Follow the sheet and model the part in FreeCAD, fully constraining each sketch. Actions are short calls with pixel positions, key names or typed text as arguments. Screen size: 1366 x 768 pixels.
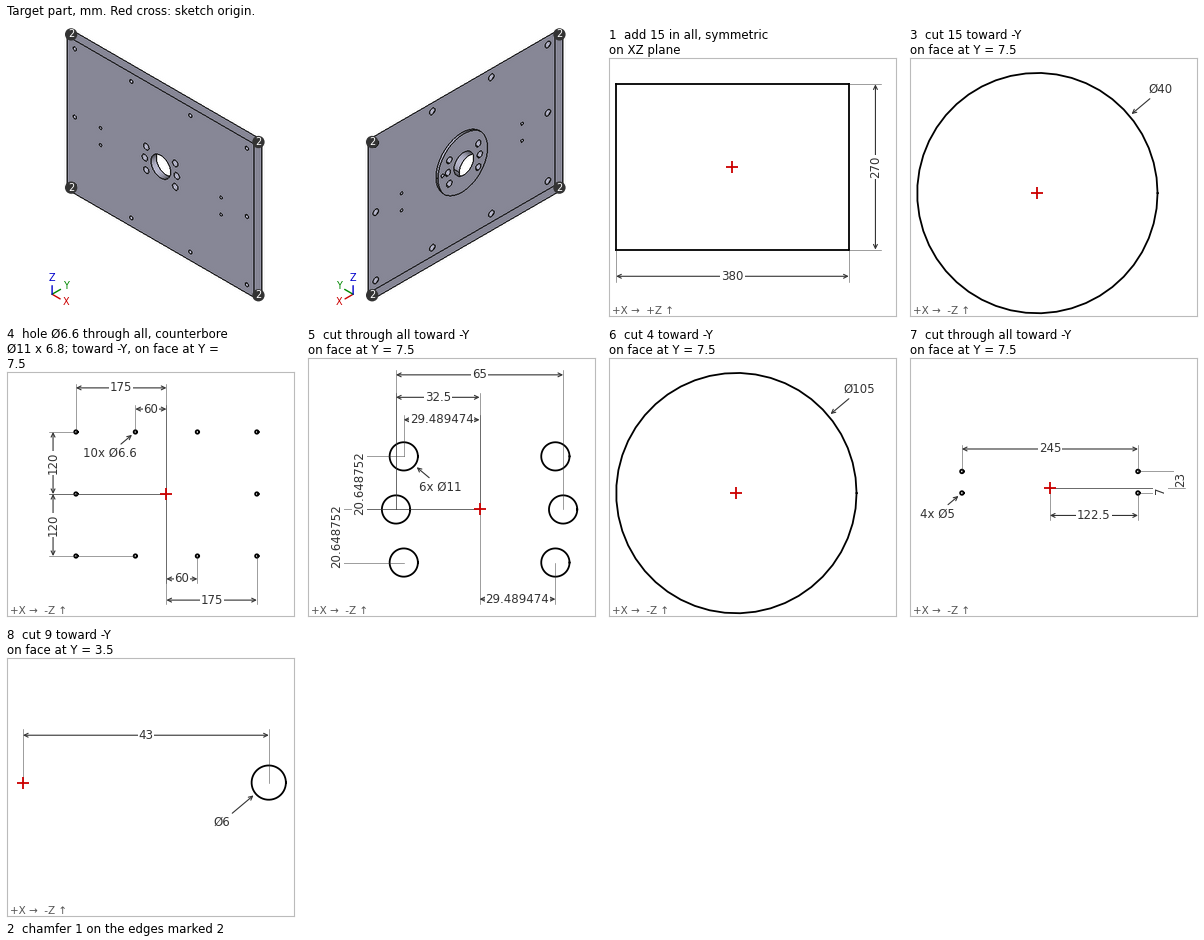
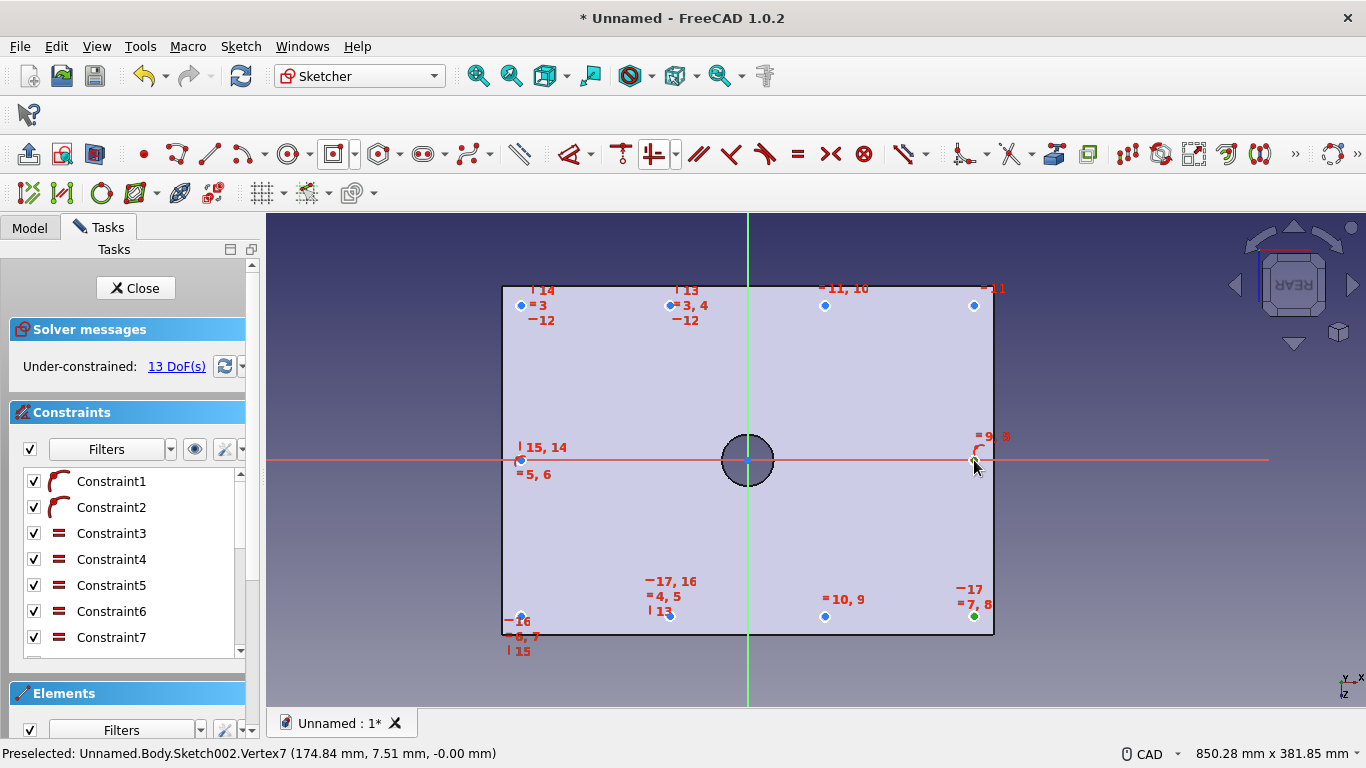
click(676, 154)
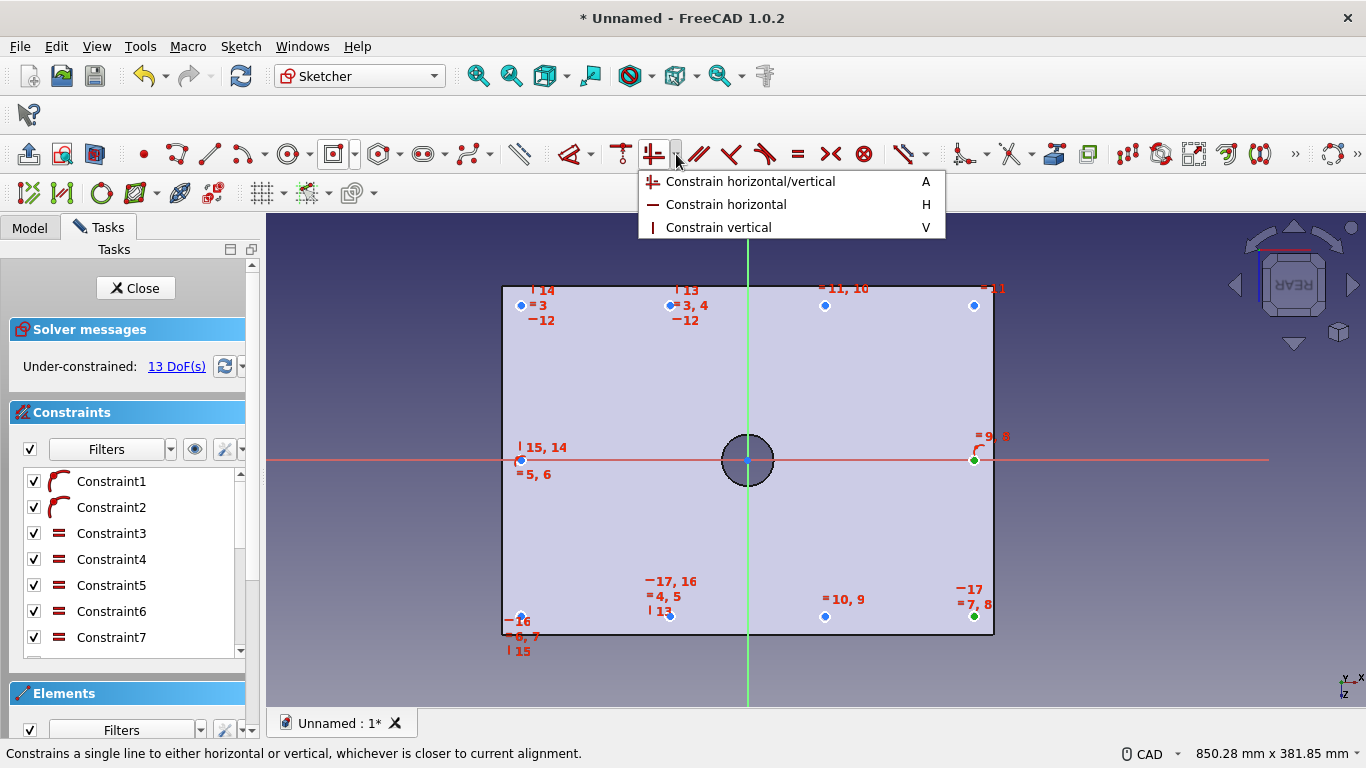
click(792, 228)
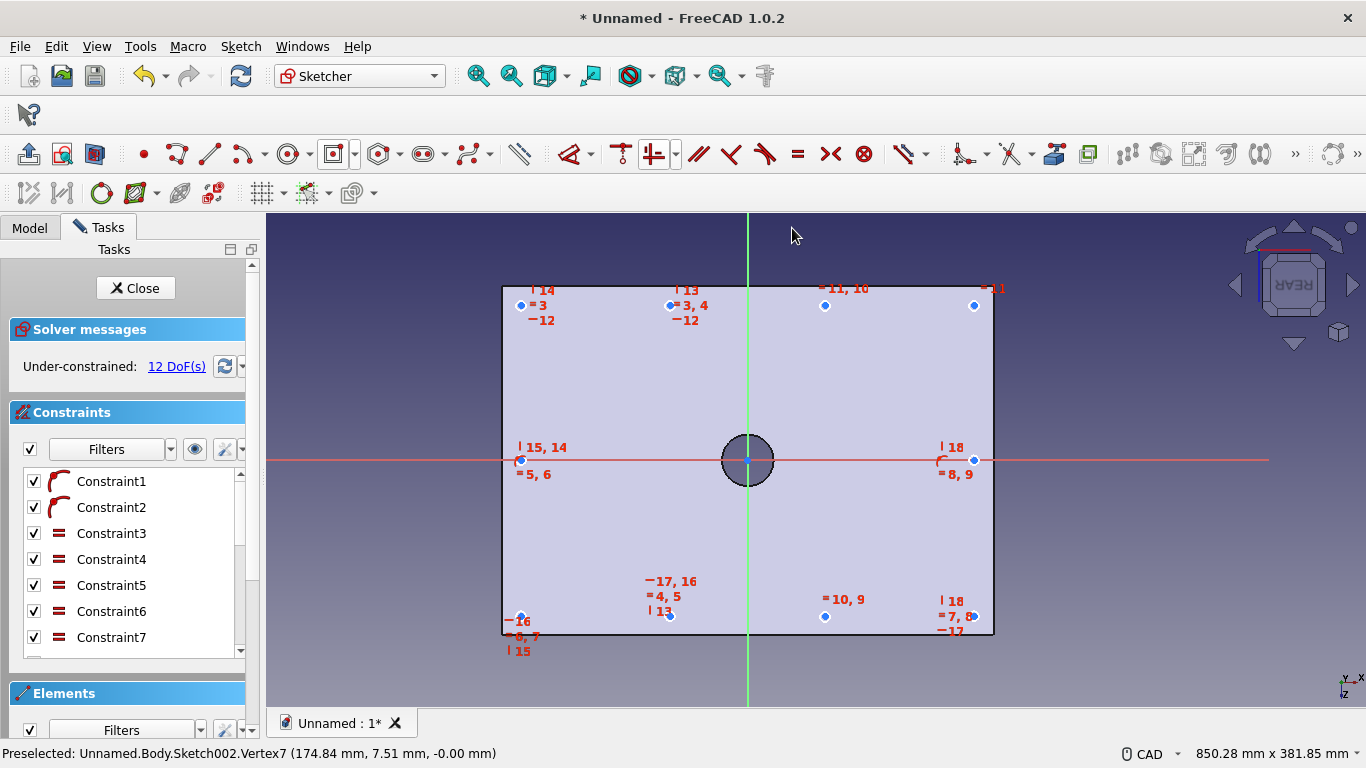
click(974, 616)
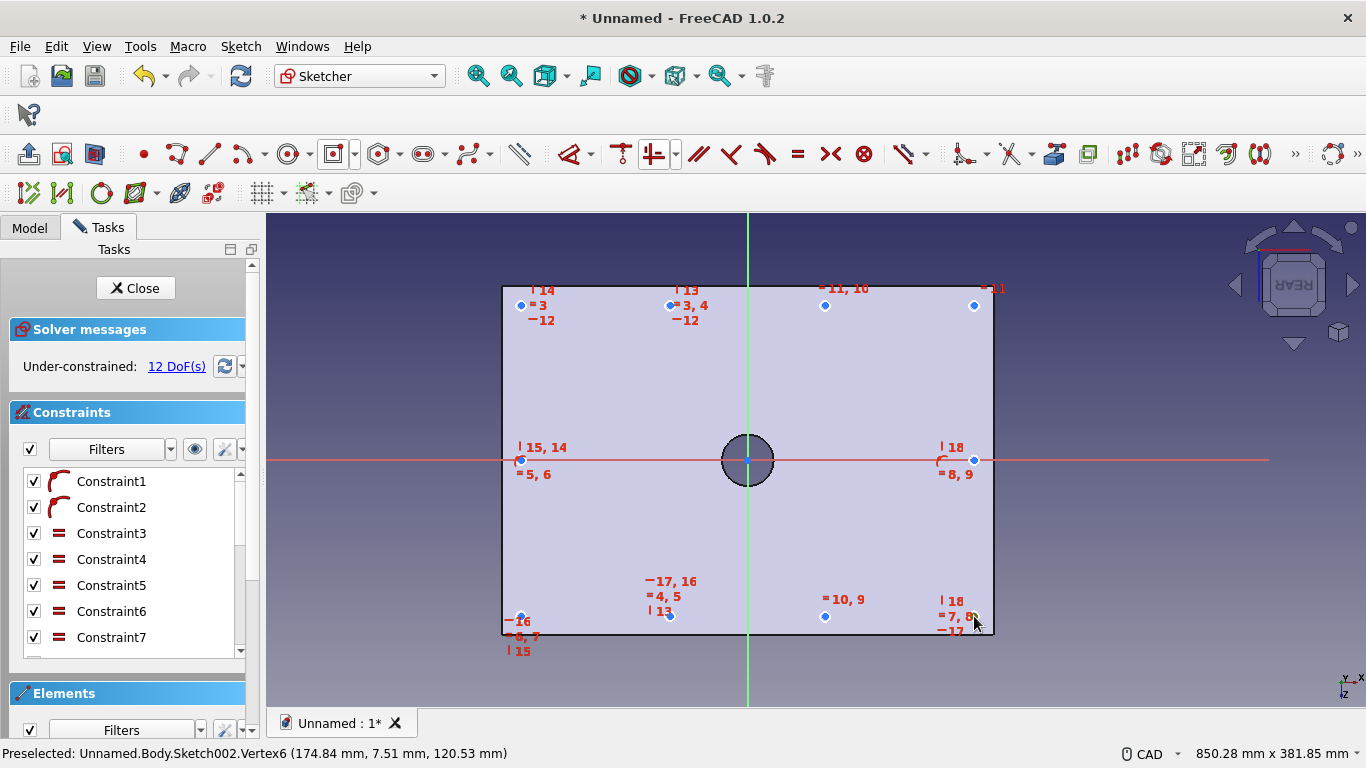
click(825, 617)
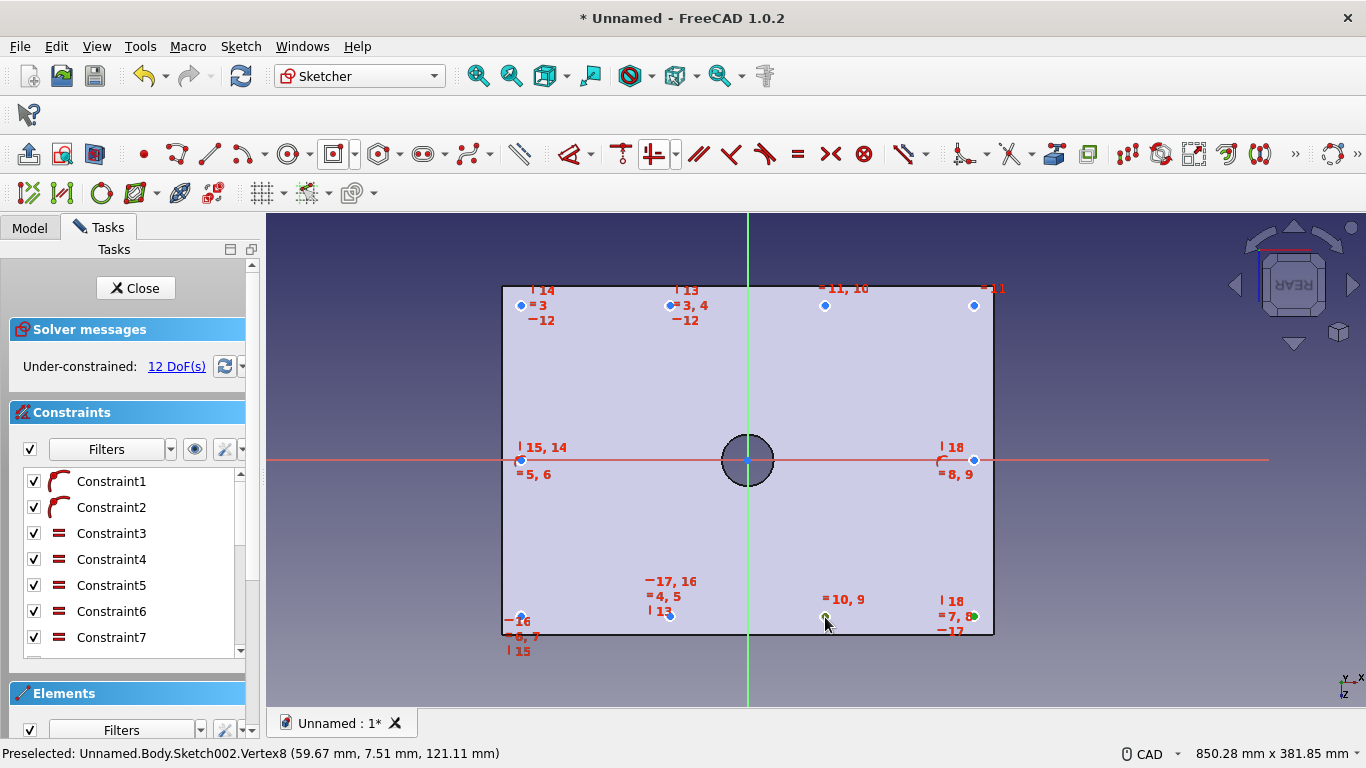
key(h)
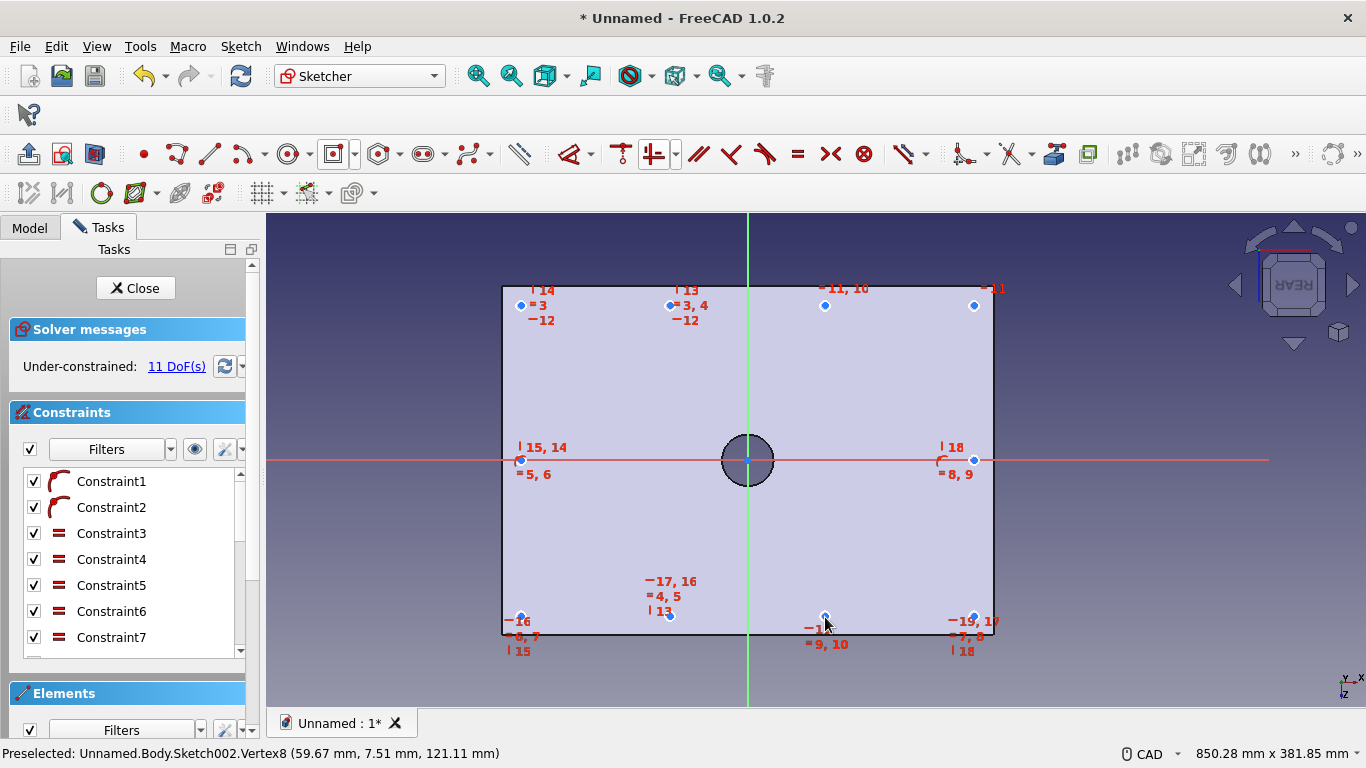
click(825, 616)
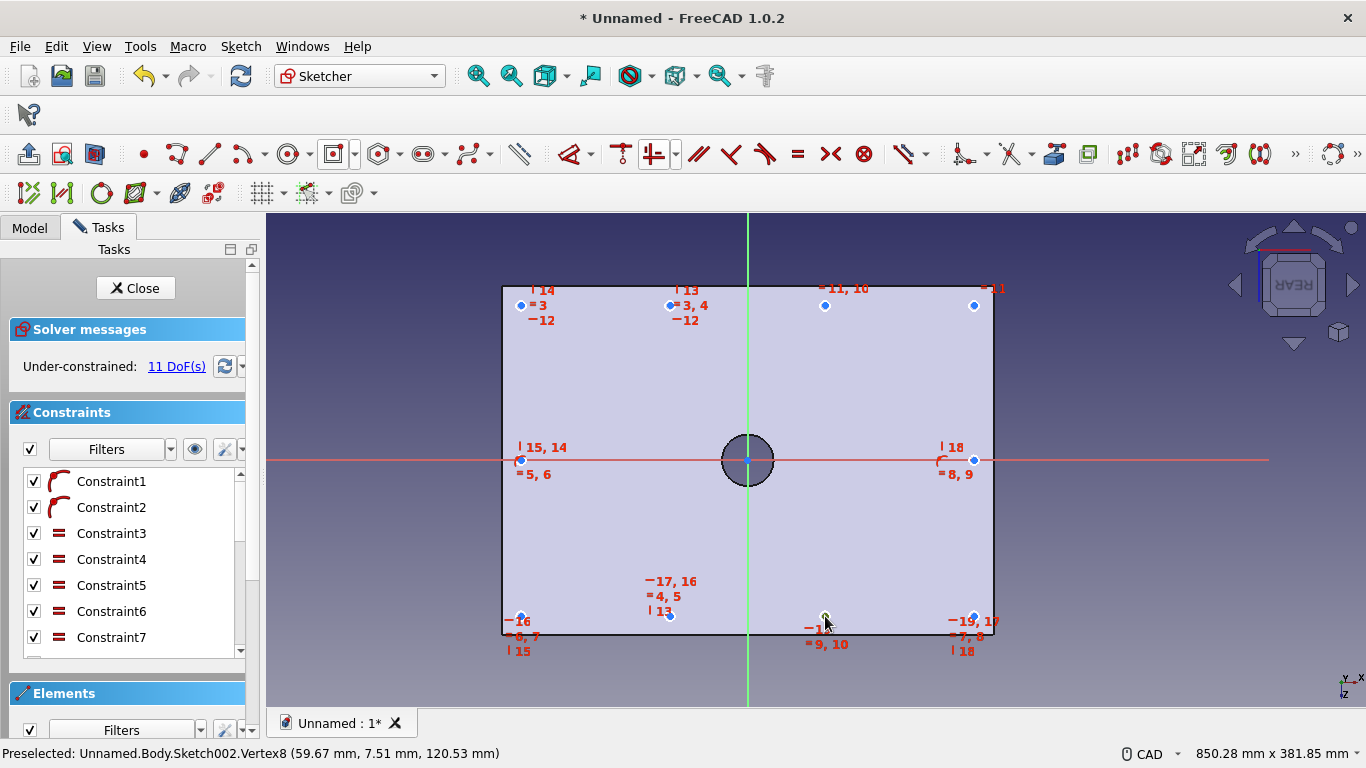
click(825, 306)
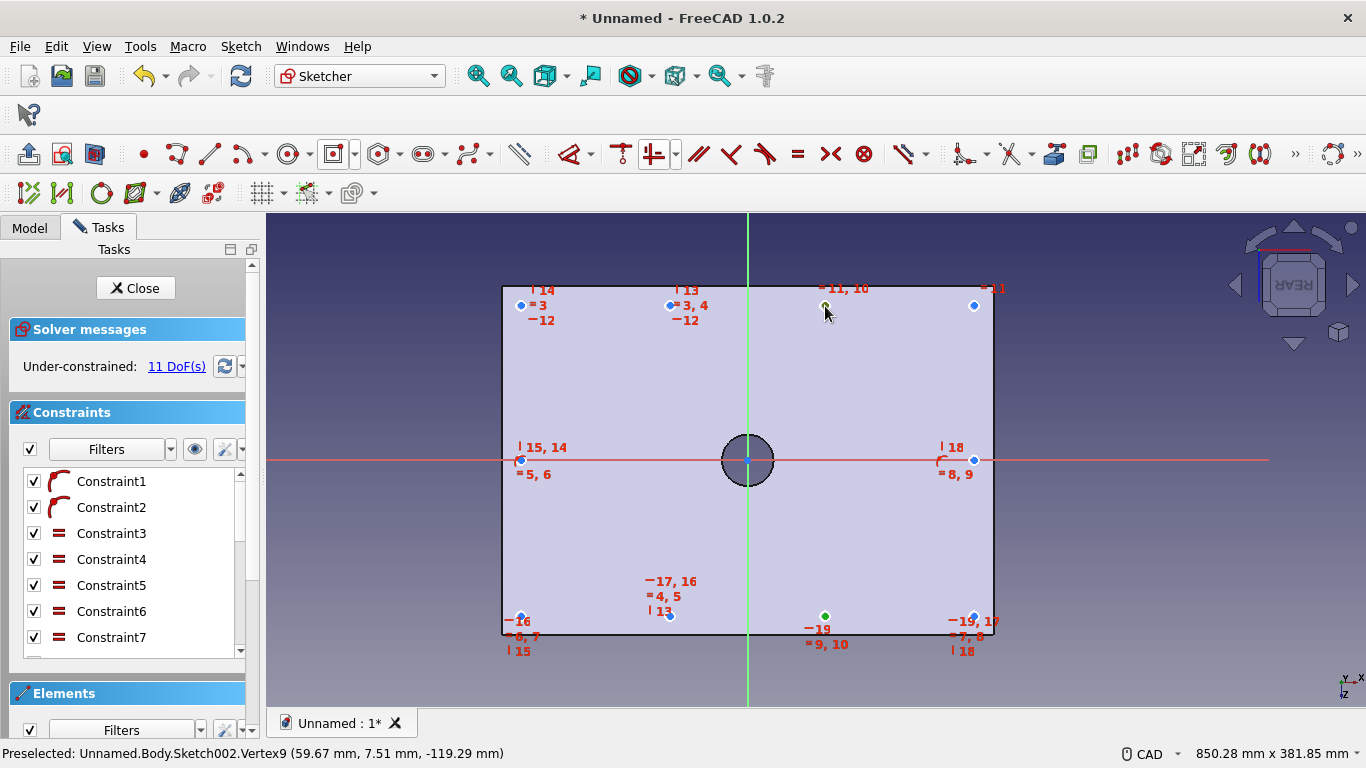
click(676, 154)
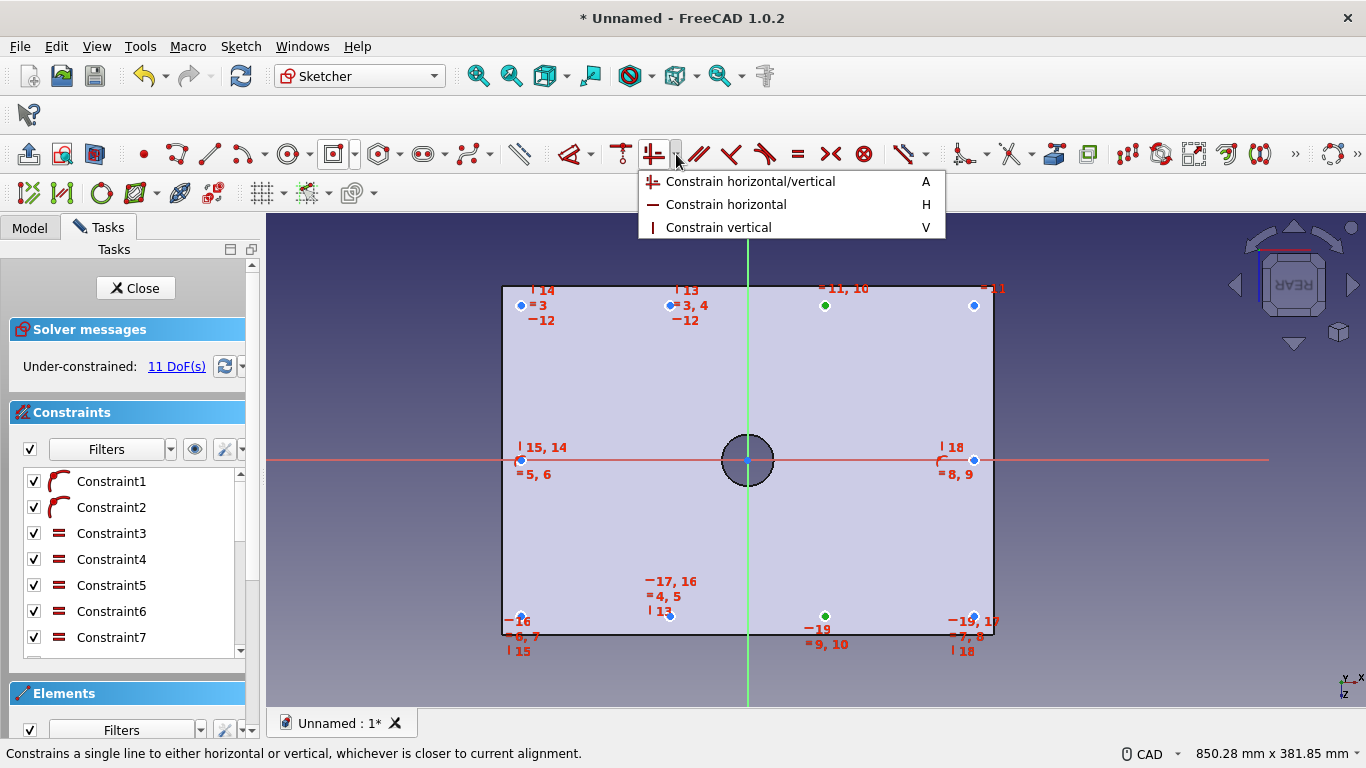
click(792, 228)